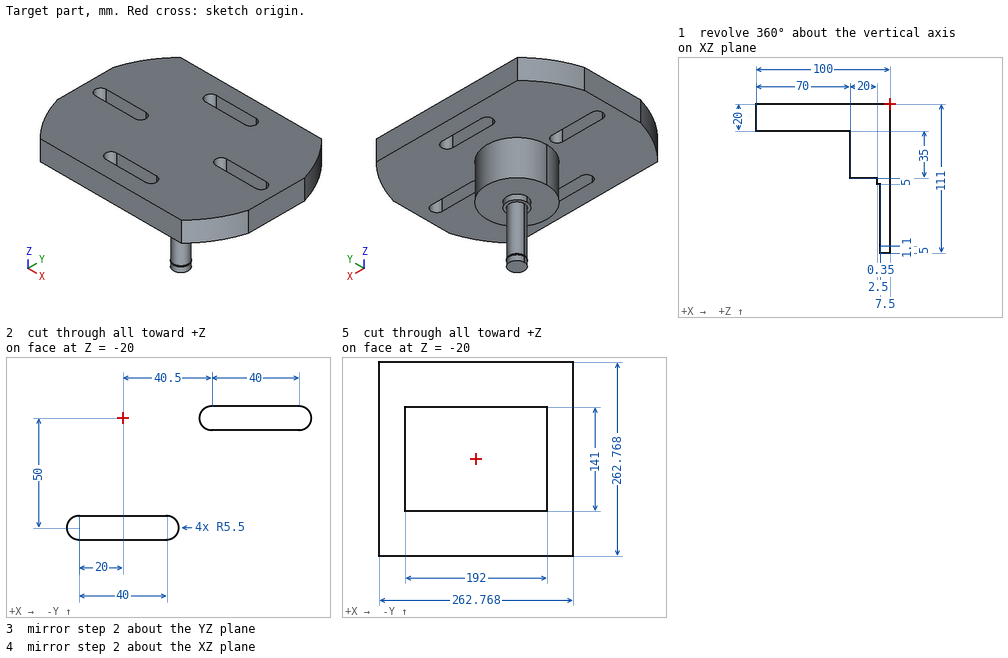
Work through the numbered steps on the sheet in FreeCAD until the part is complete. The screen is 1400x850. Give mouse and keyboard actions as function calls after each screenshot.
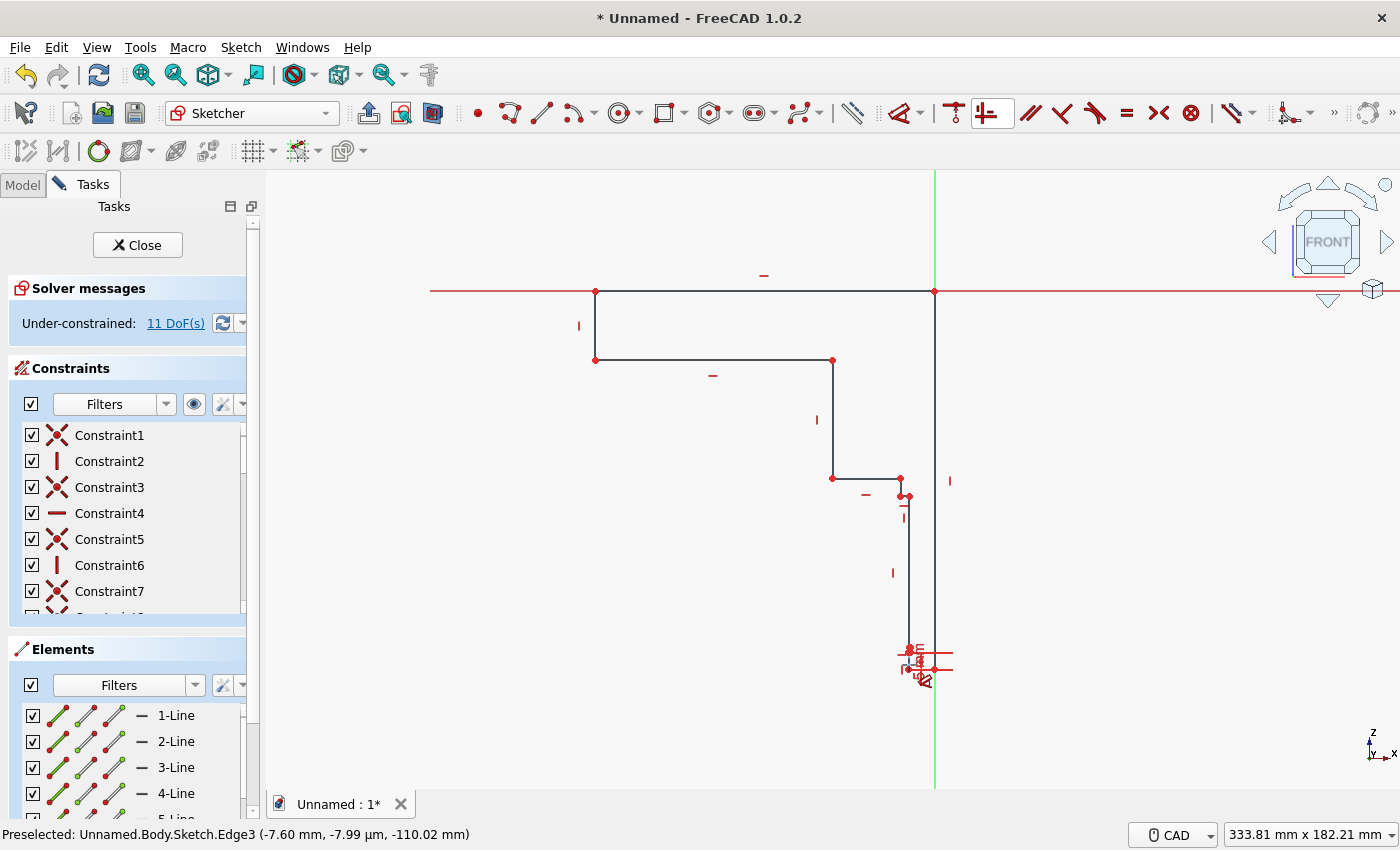
scroll(901, 491, up, 5)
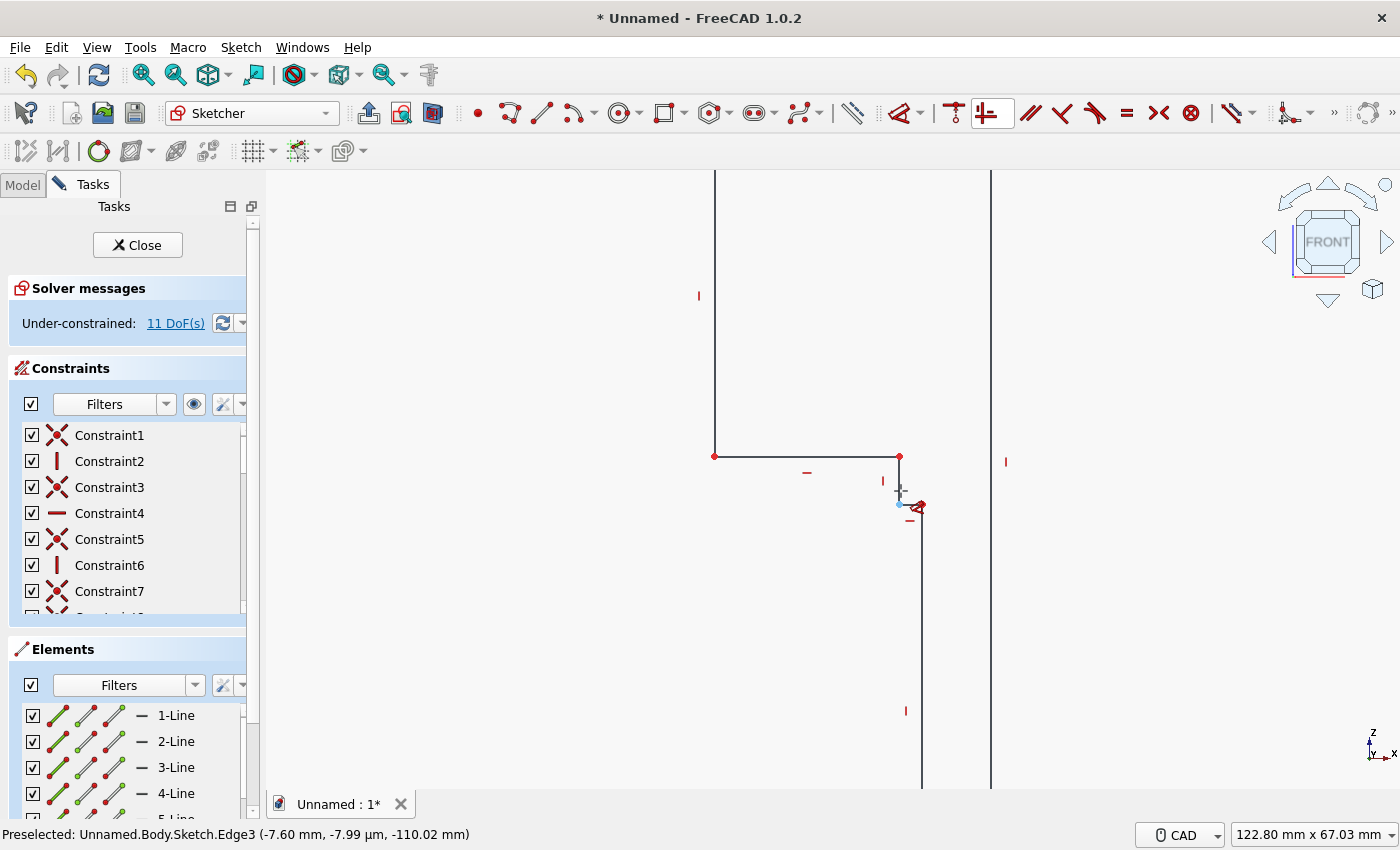
click(899, 490)
click(933, 481)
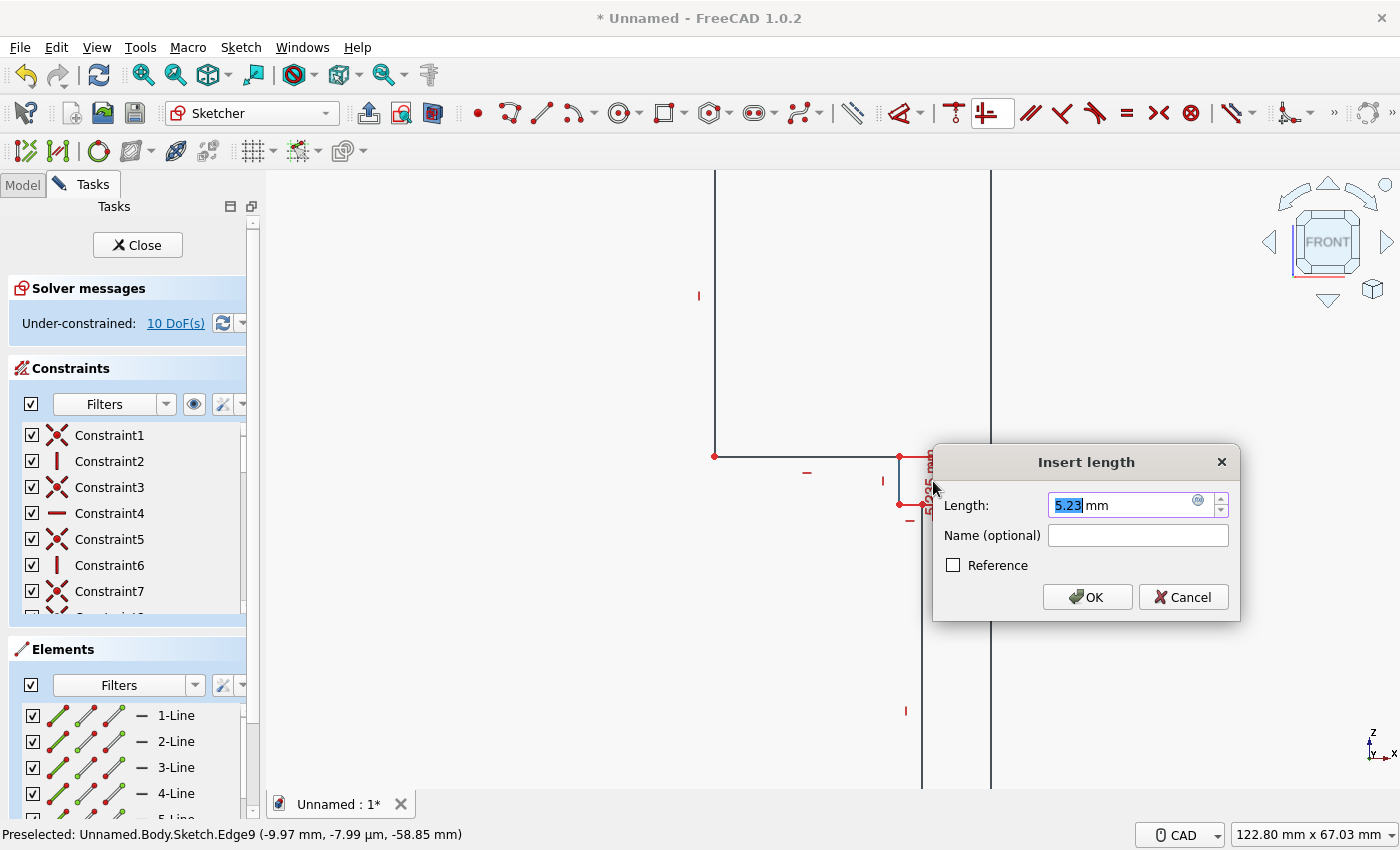
text(5)
key(Return)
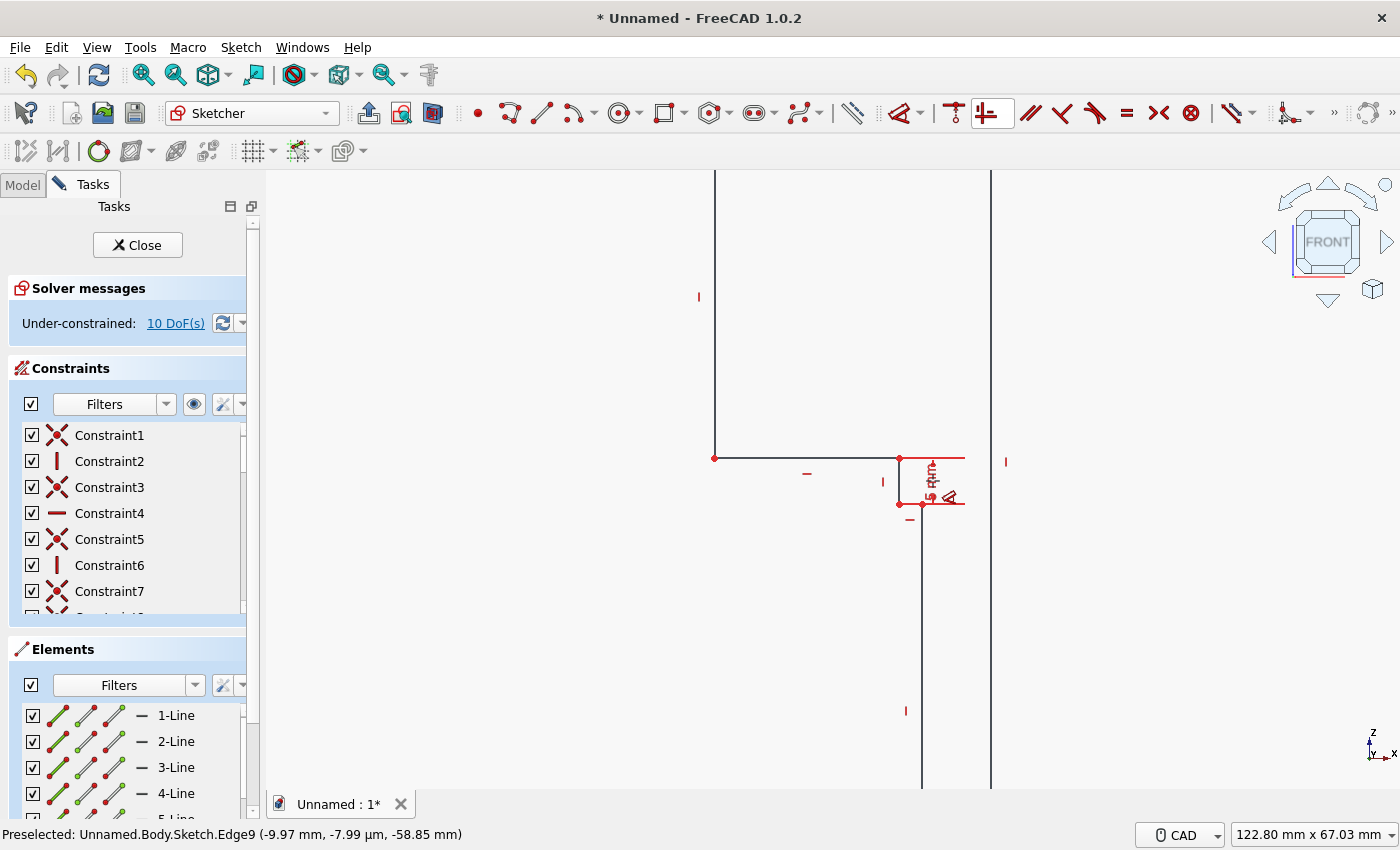
click(844, 458)
click(807, 424)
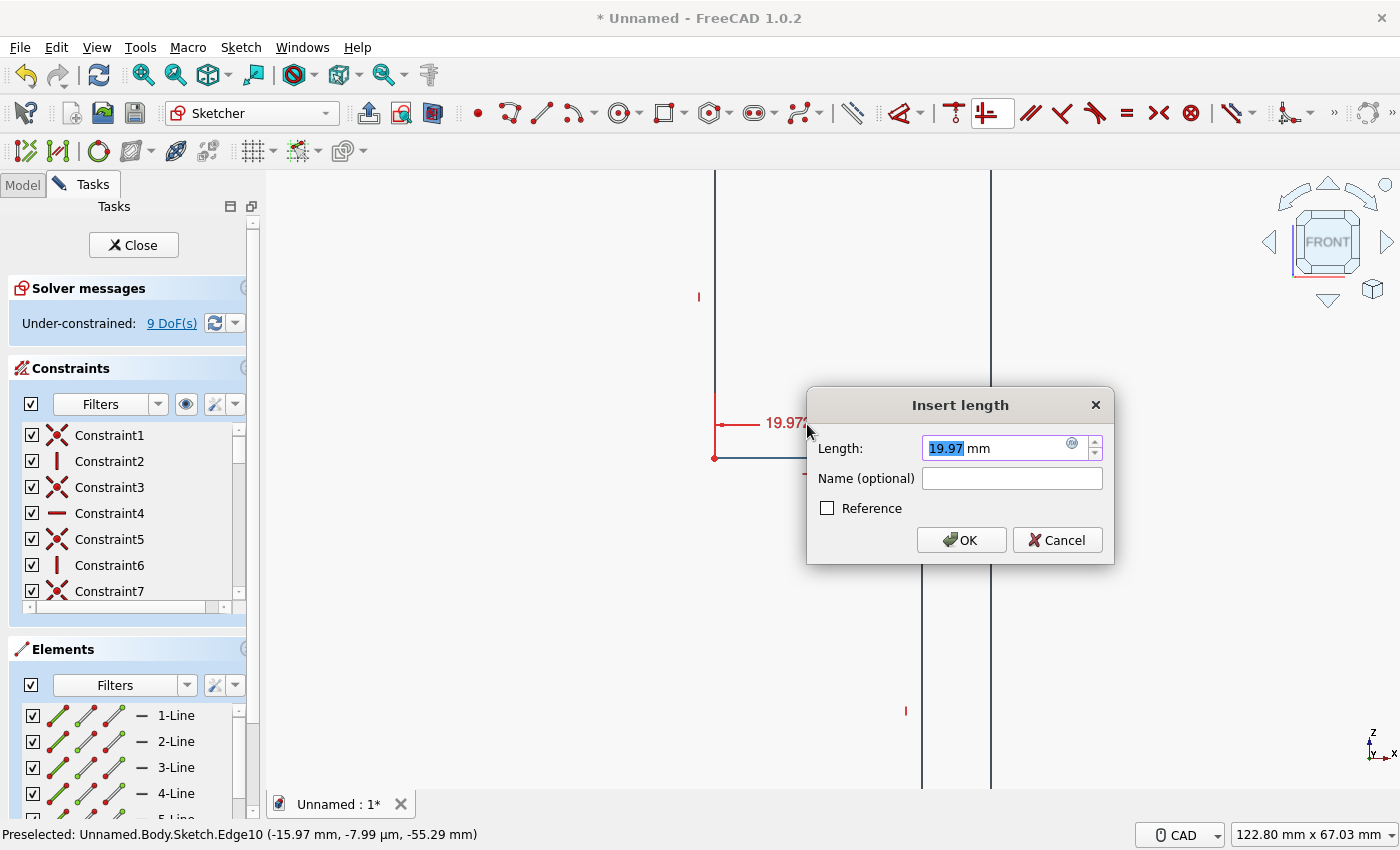
text(20)
key(Return)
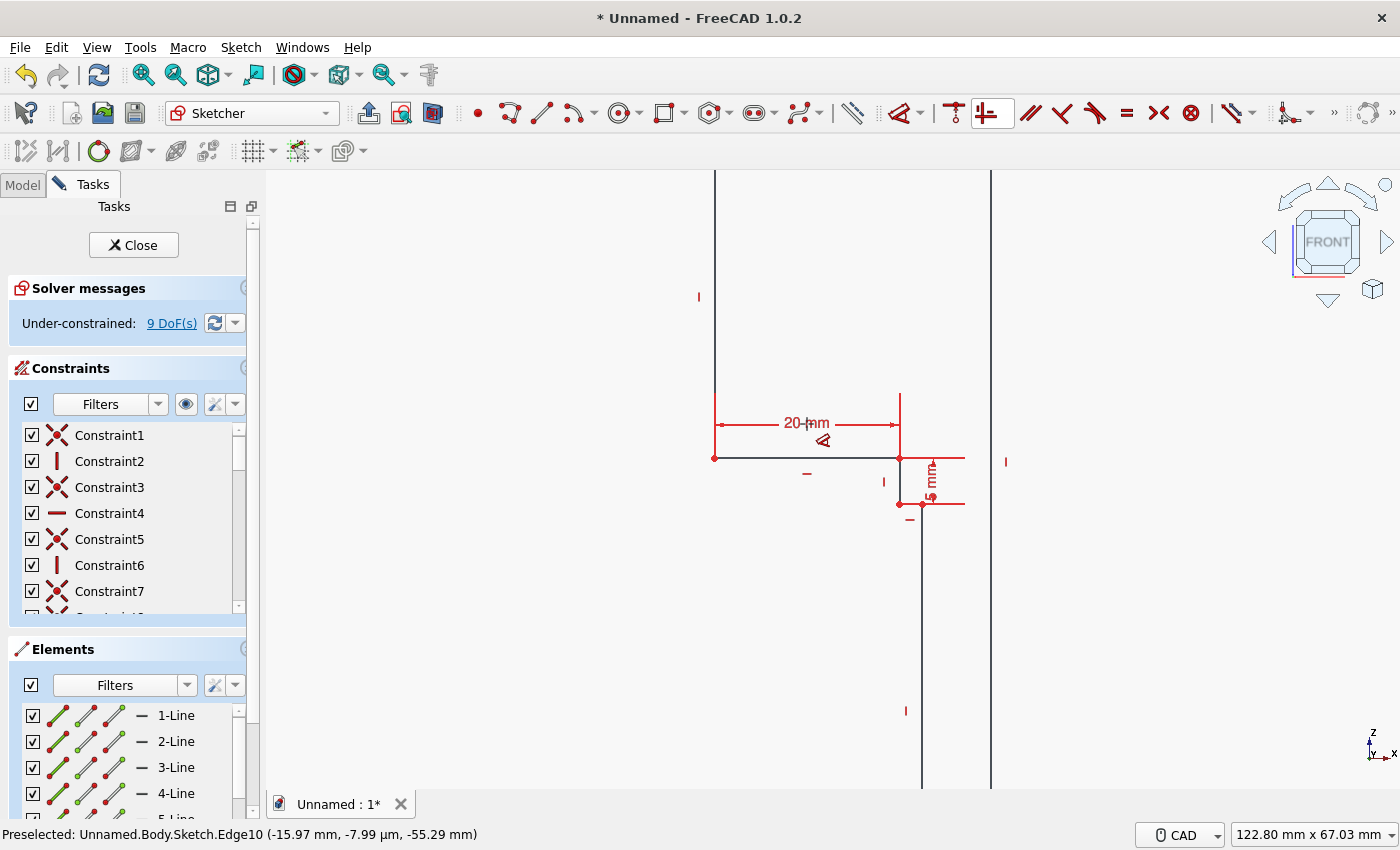
click(715, 361)
click(749, 328)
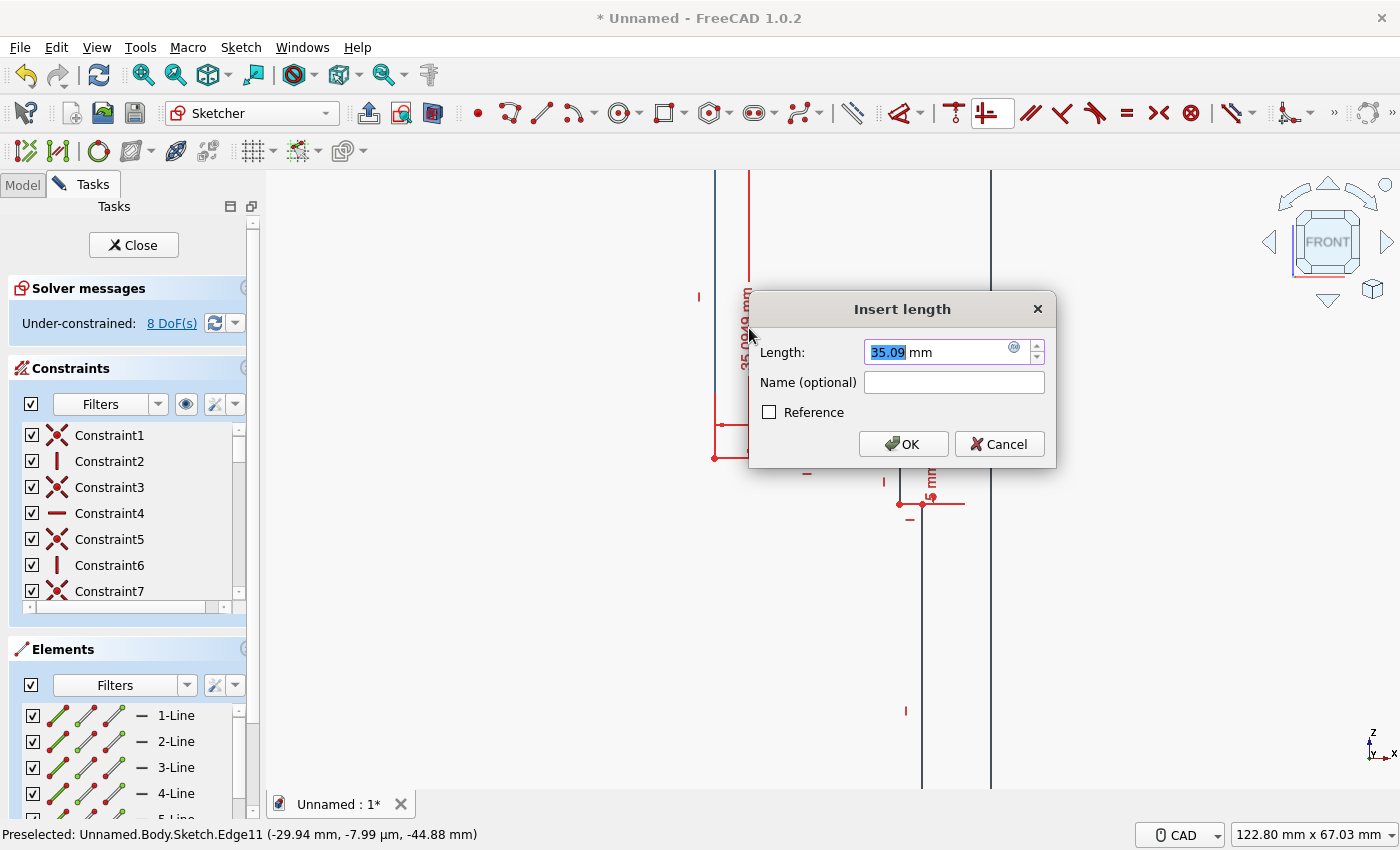
text(35)
key(Return)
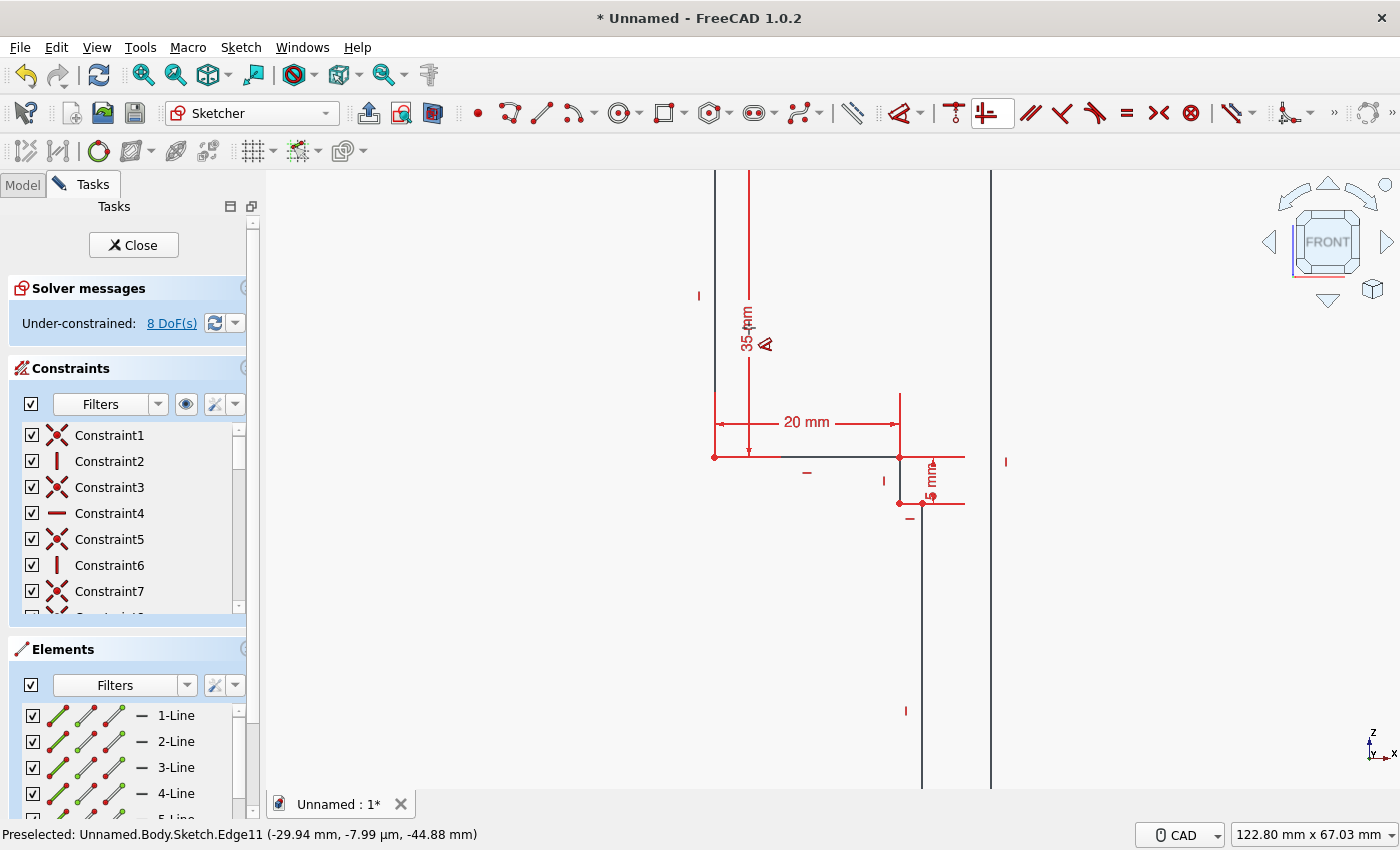
scroll(901, 491, down, 5)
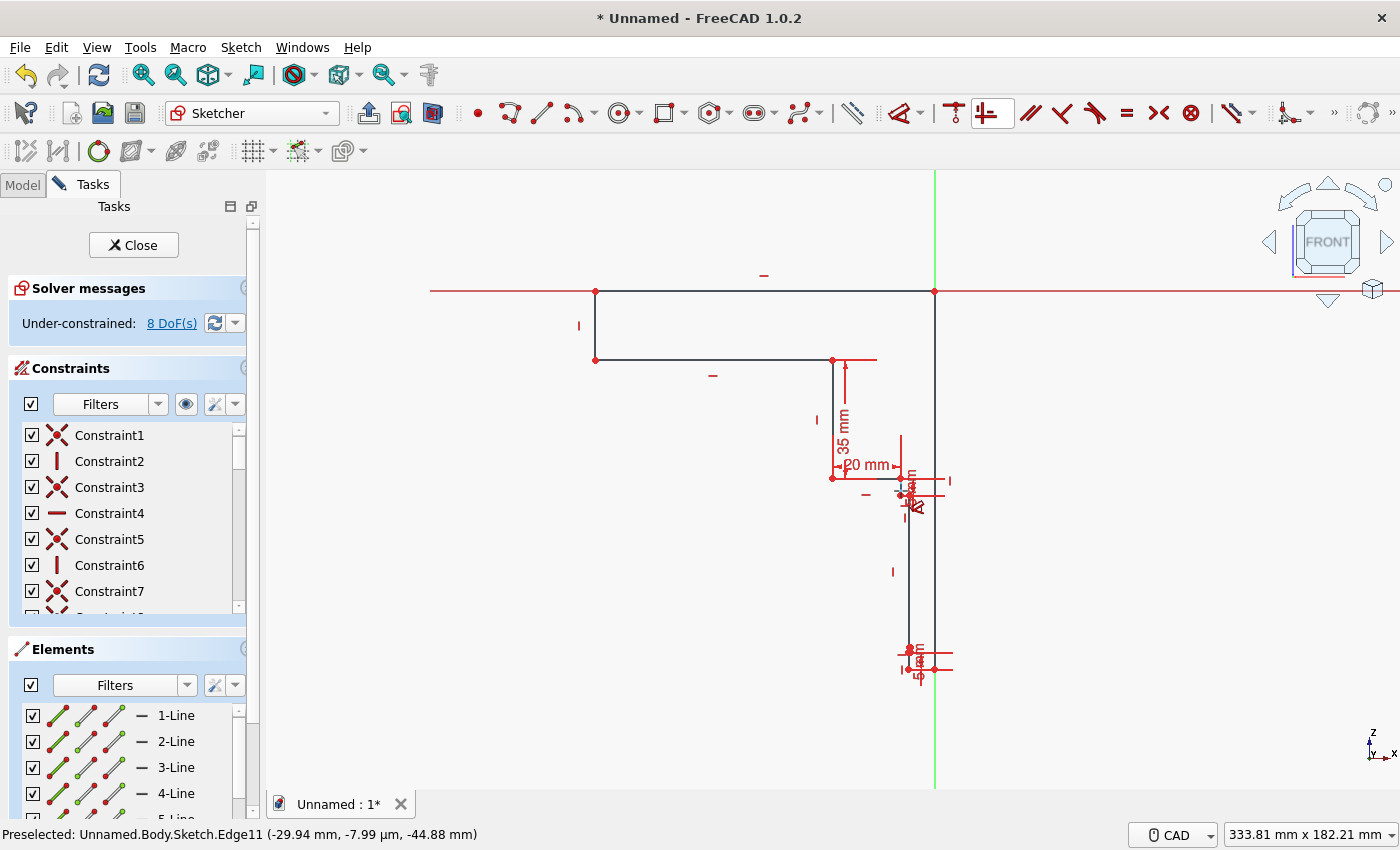
click(762, 360)
click(714, 326)